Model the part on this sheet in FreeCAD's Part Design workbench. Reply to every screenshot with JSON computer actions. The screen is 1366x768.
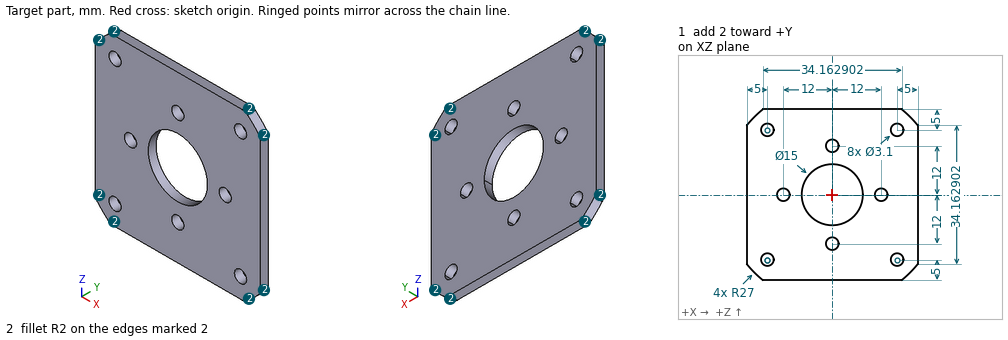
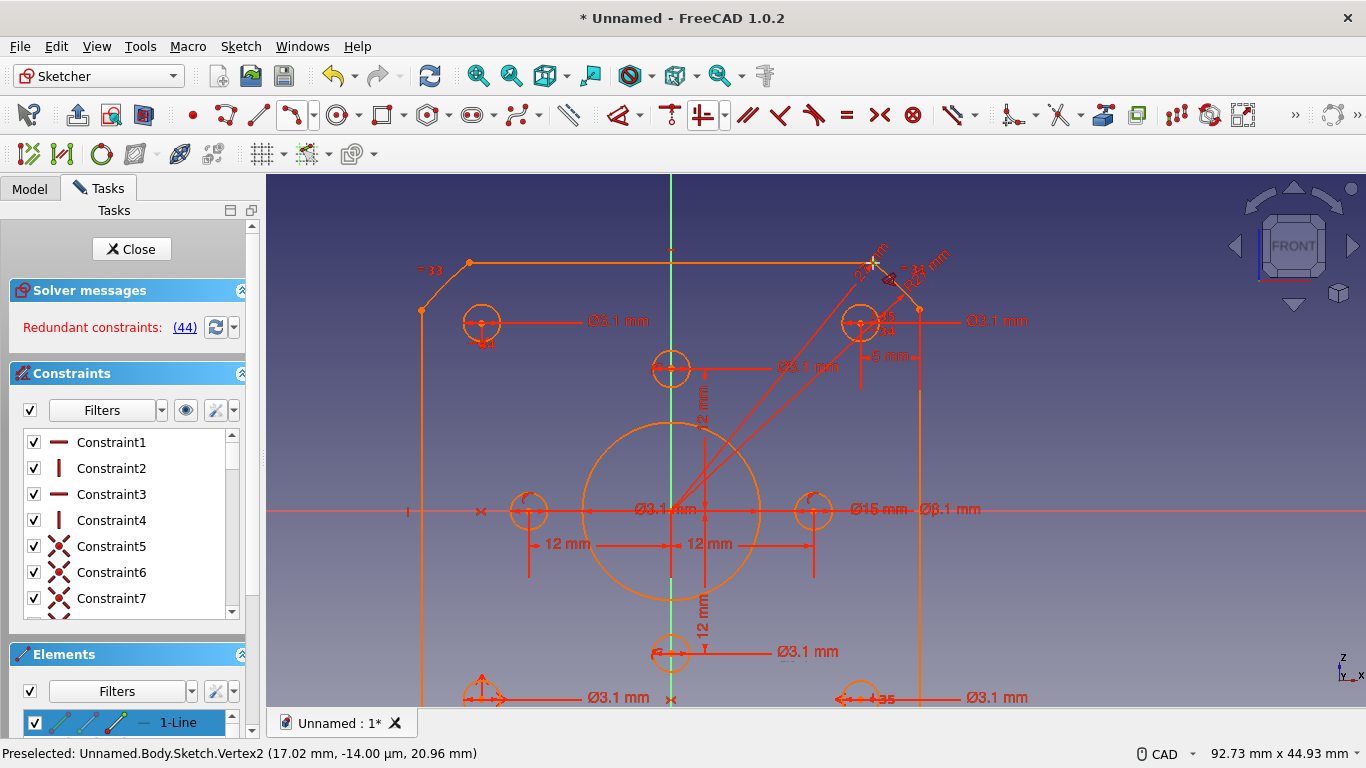
{"action": "left_click", "coordinate": [861, 323]}
{"action": "left_click", "coordinate": [827, 293]}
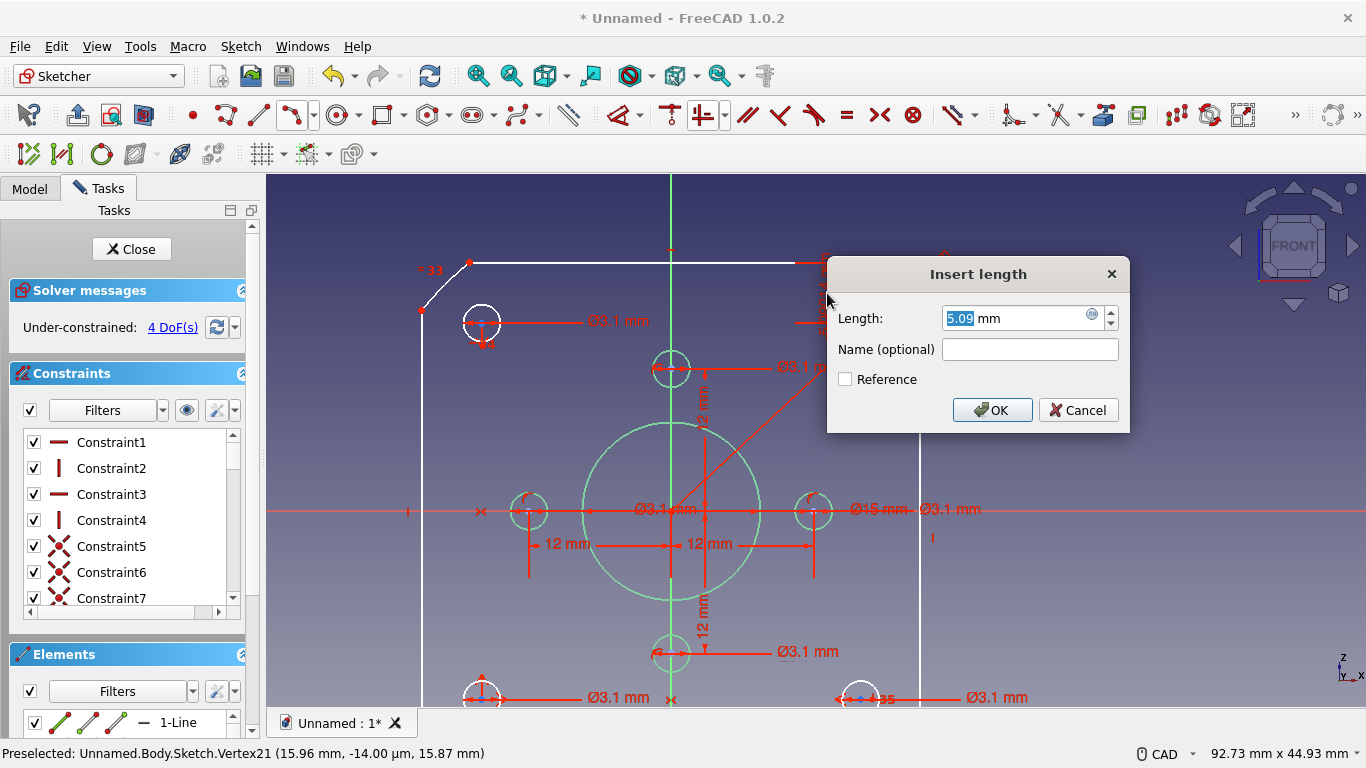
{"action": "type", "text": "5"}
{"action": "key", "text": "Return"}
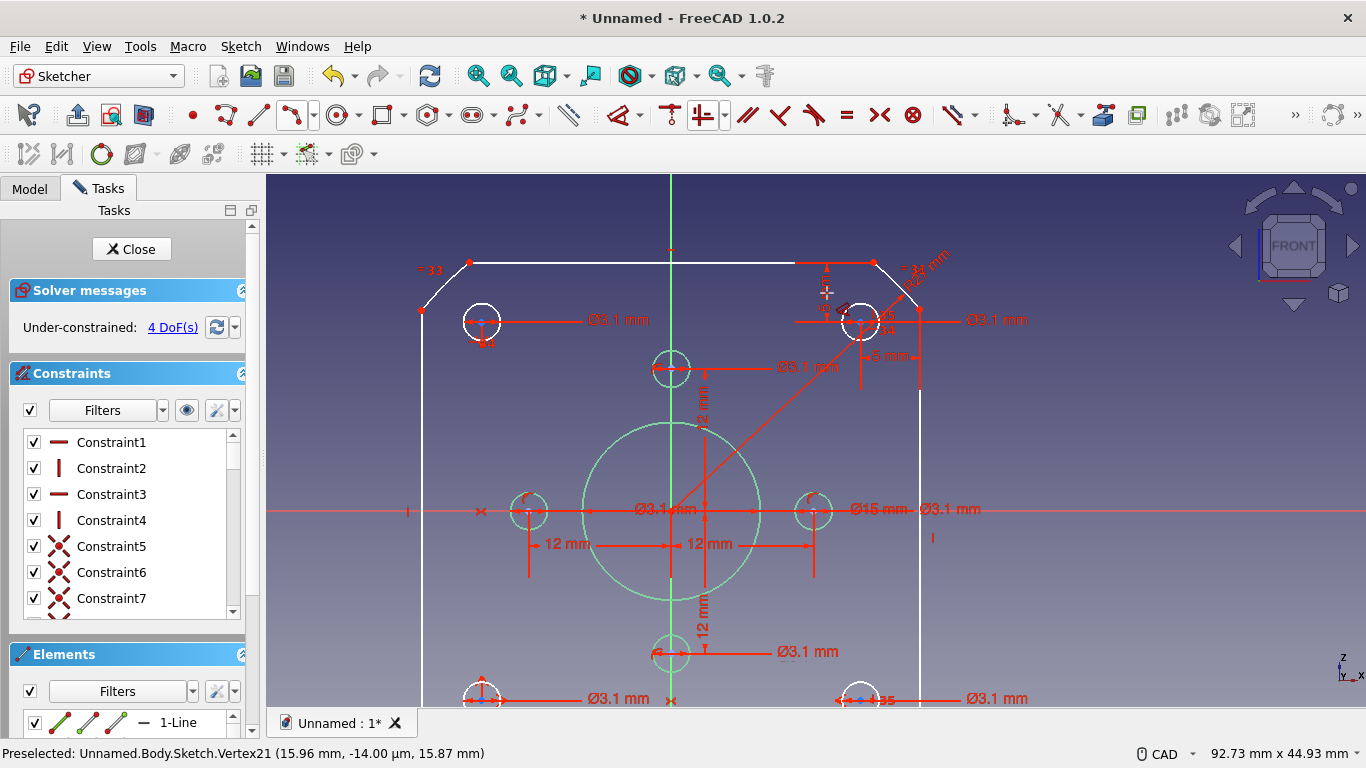
{"action": "left_click", "coordinate": [422, 310]}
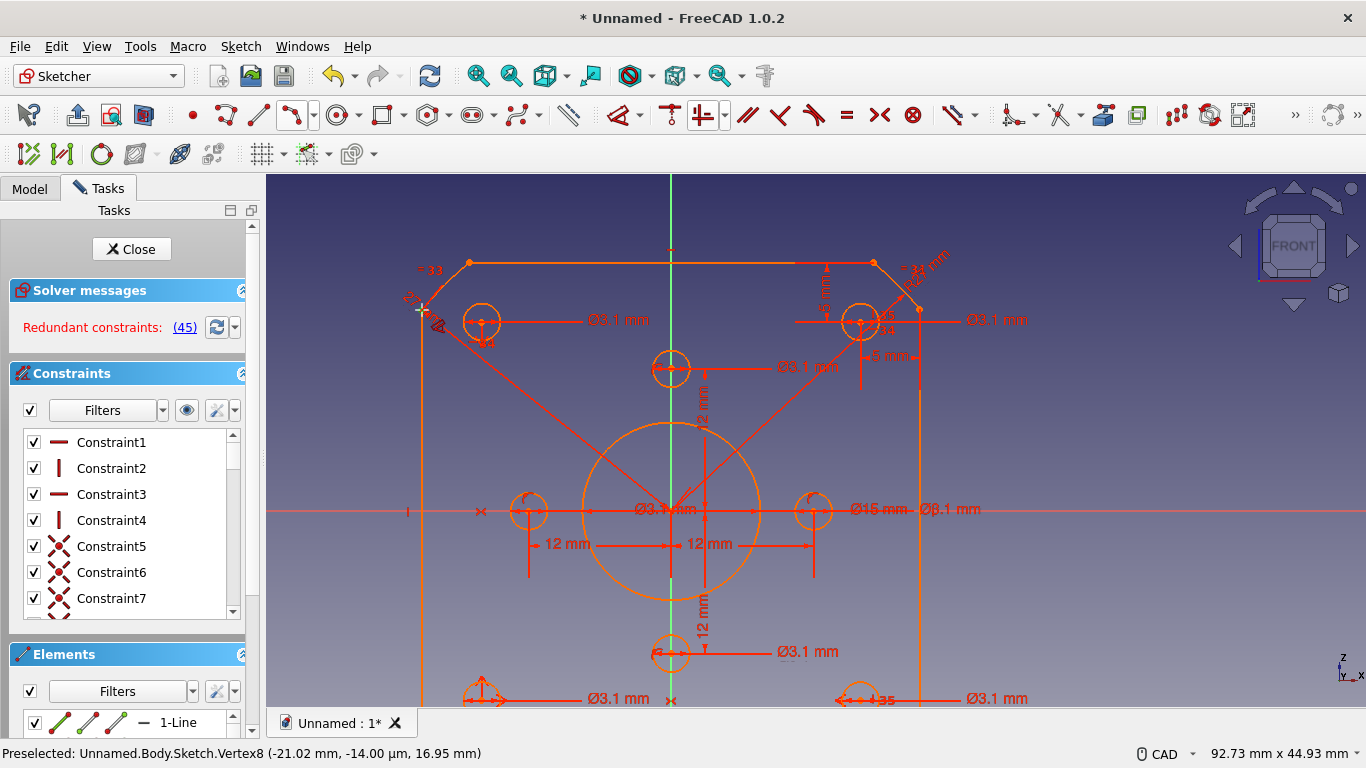
{"action": "left_click", "coordinate": [482, 322]}
{"action": "left_click", "coordinate": [431, 276]}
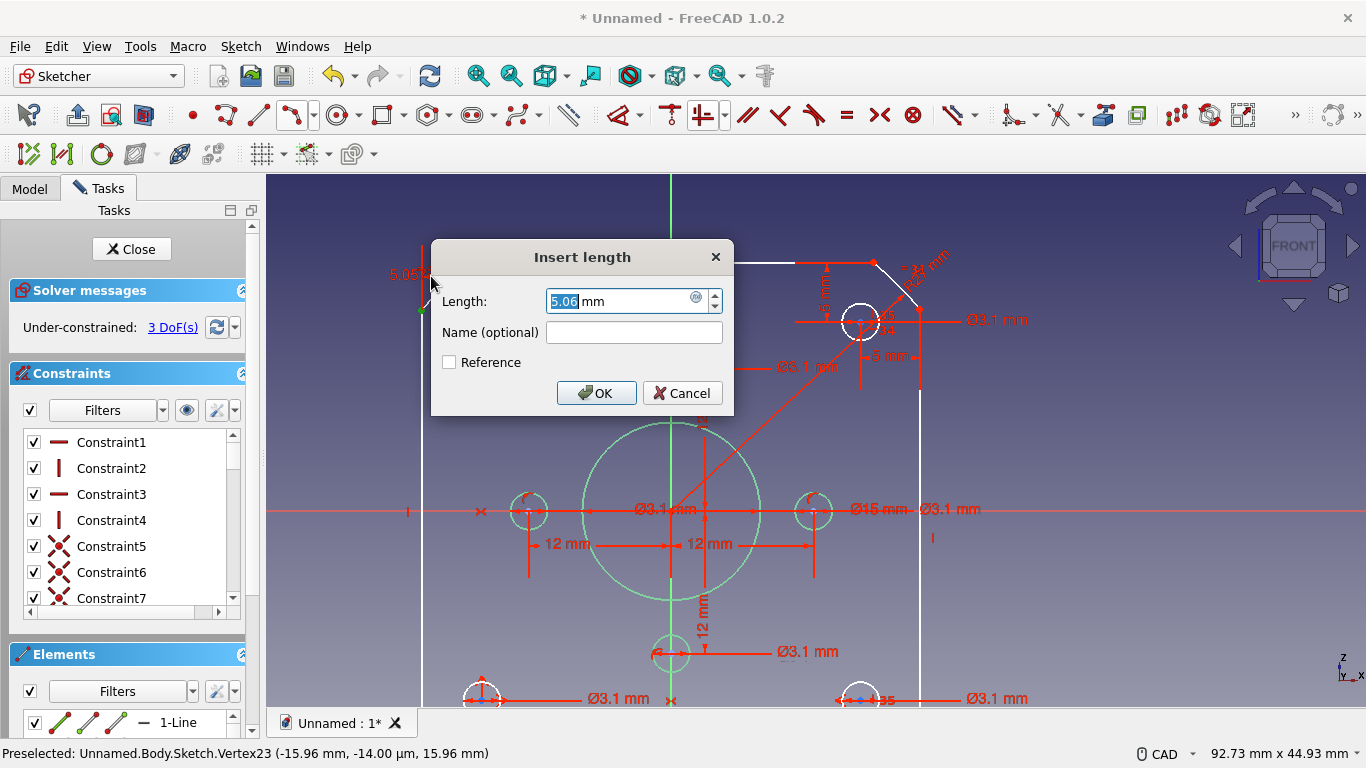
{"action": "type", "text": "5"}
{"action": "key", "text": "Return"}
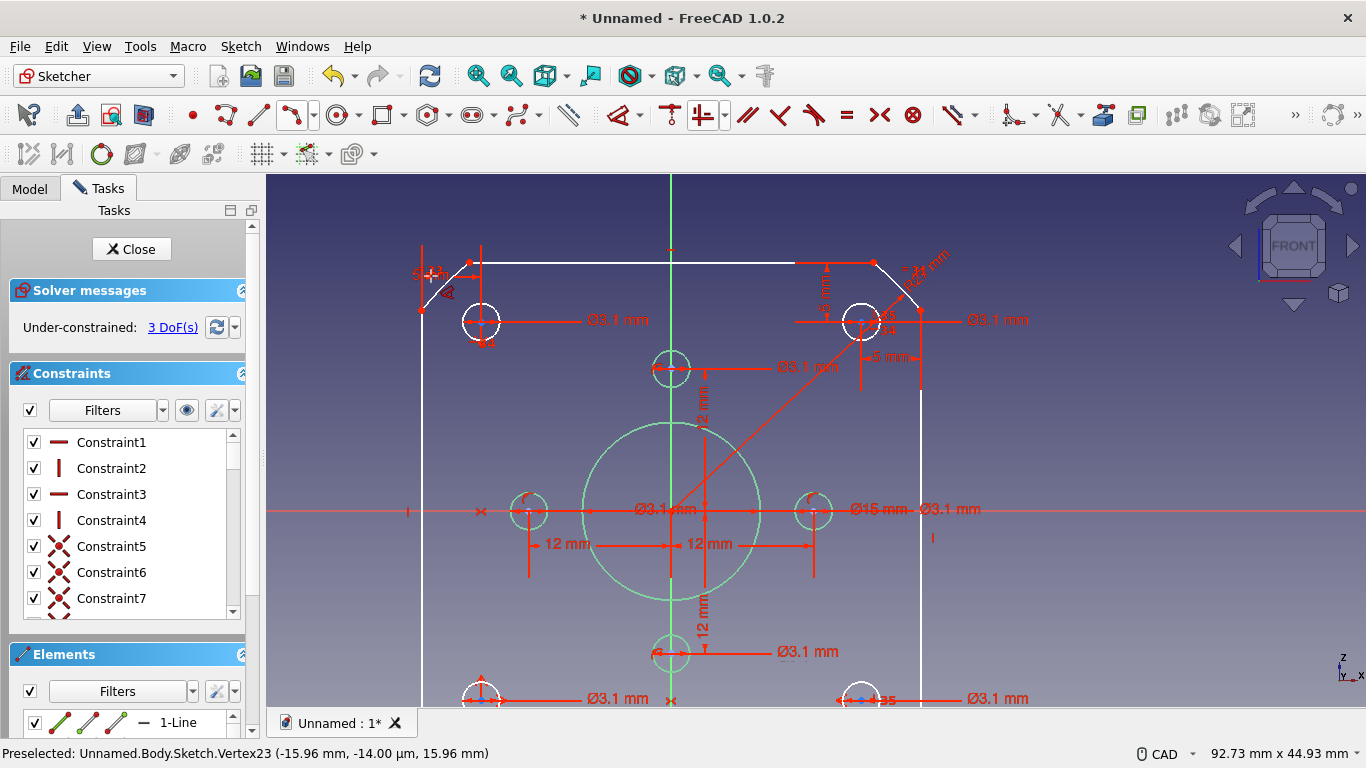
{"action": "scroll", "coordinate": [902, 297], "scroll_direction": "down", "scroll_amount": 2}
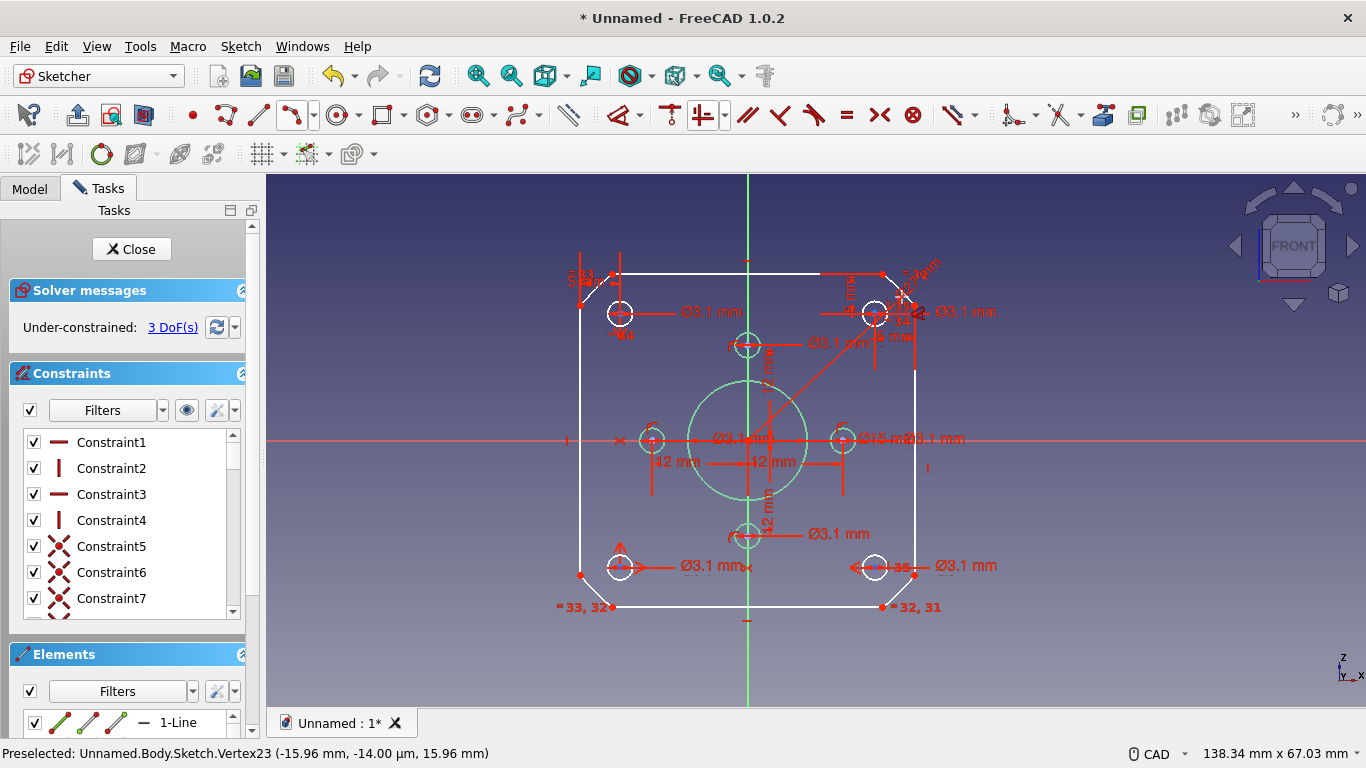
{"action": "left_click", "coordinate": [883, 607]}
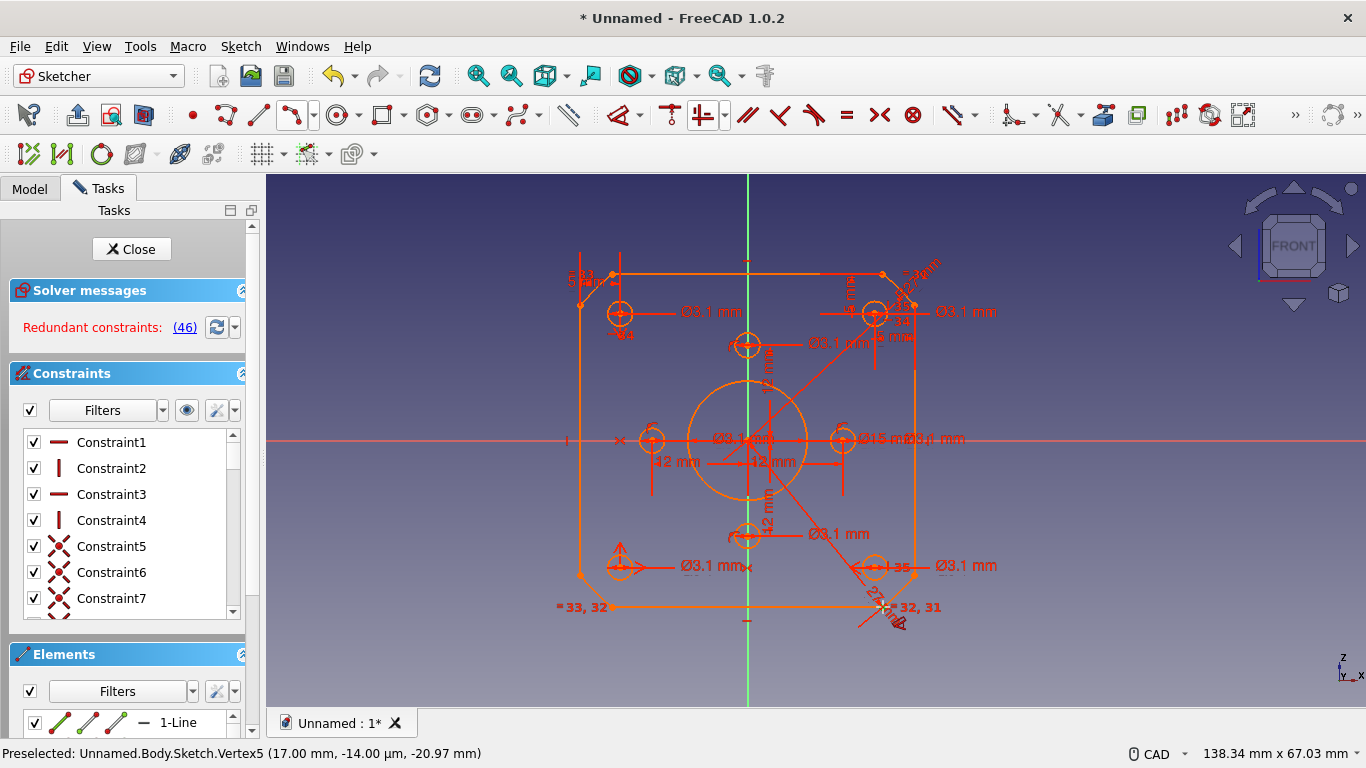
{"action": "left_click", "coordinate": [875, 568]}
{"action": "left_click", "coordinate": [917, 597]}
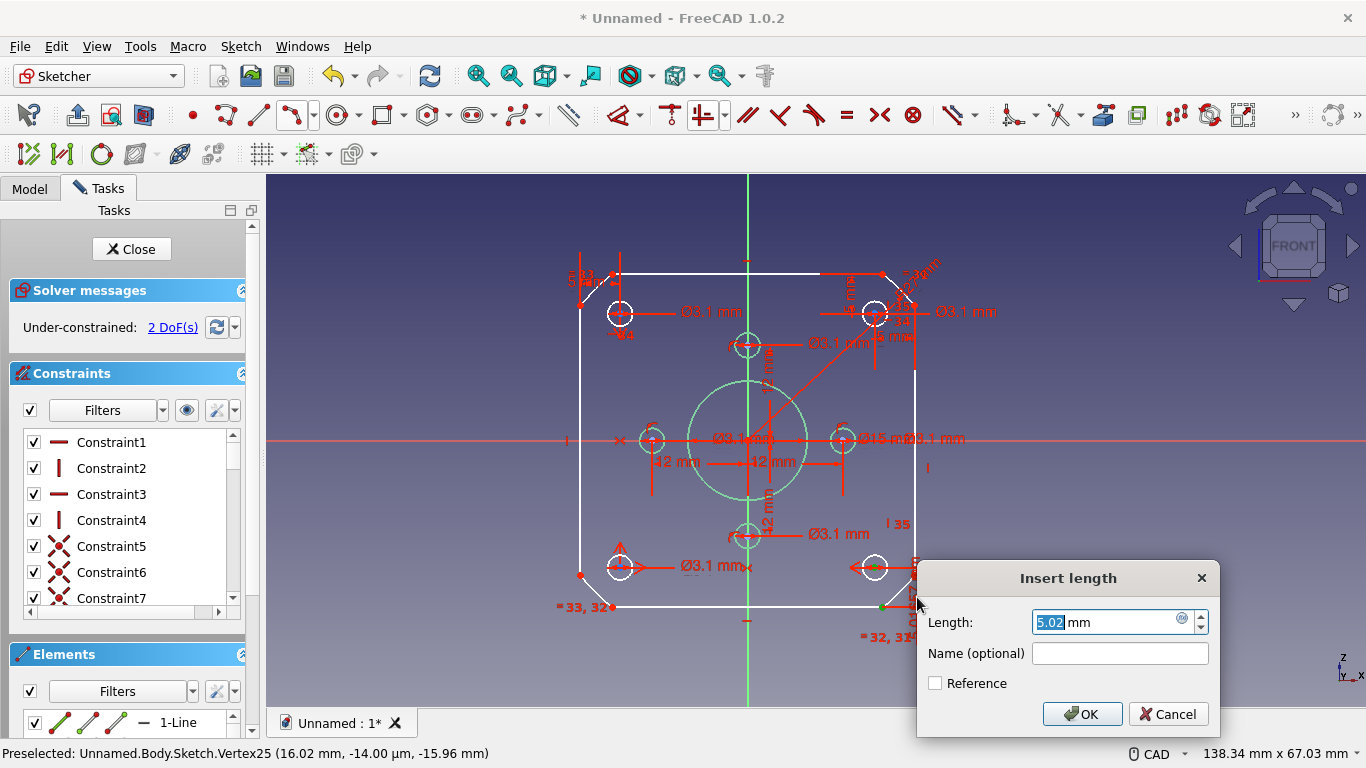
{"action": "type", "text": "5"}
{"action": "key", "text": "Return"}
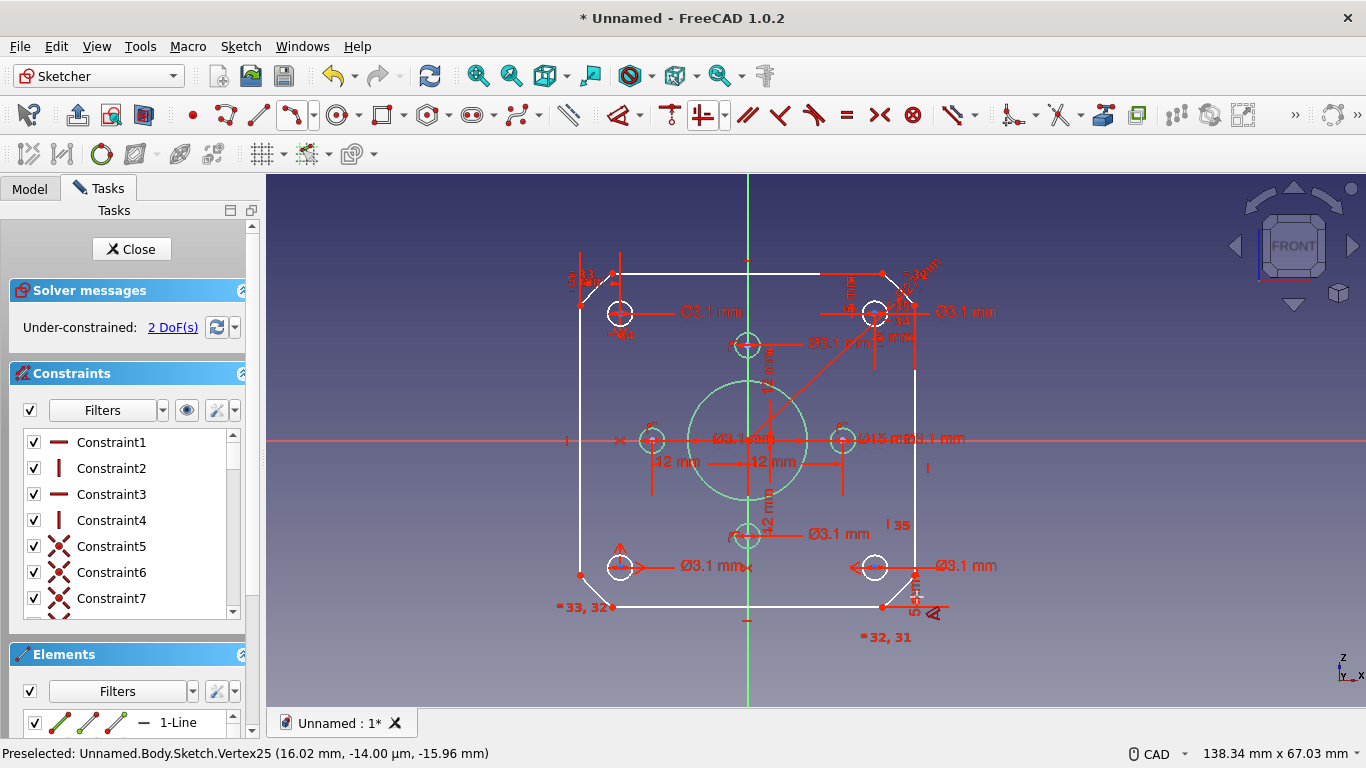
{"action": "left_click", "coordinate": [693, 274]}
{"action": "left_click", "coordinate": [685, 240]}